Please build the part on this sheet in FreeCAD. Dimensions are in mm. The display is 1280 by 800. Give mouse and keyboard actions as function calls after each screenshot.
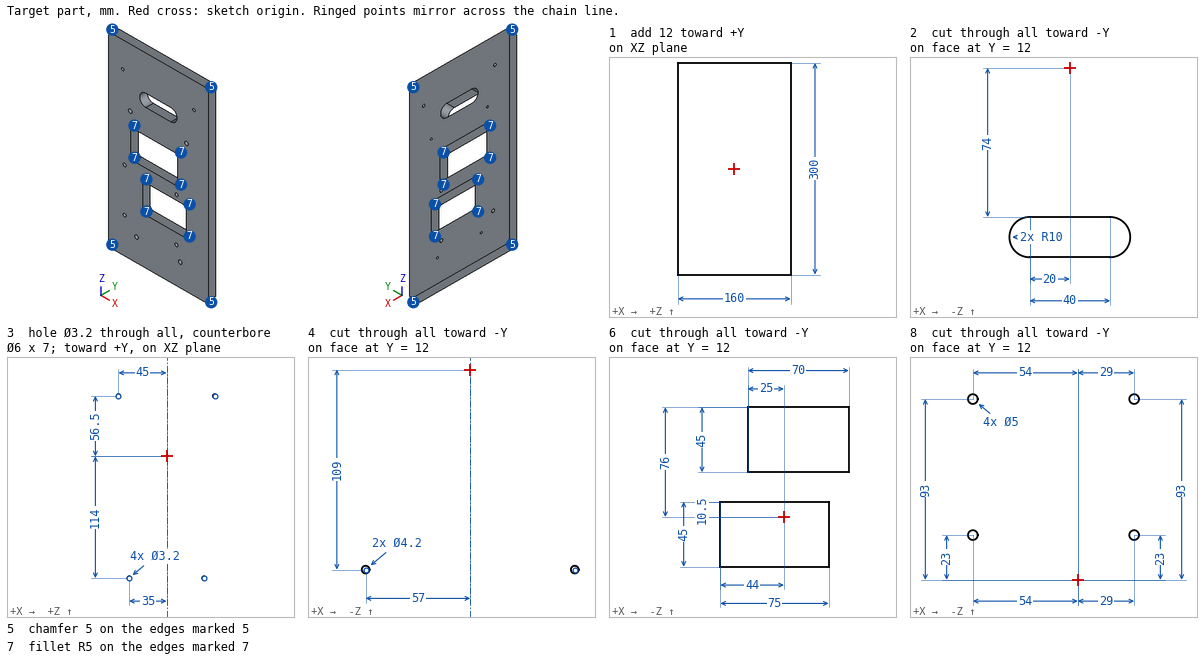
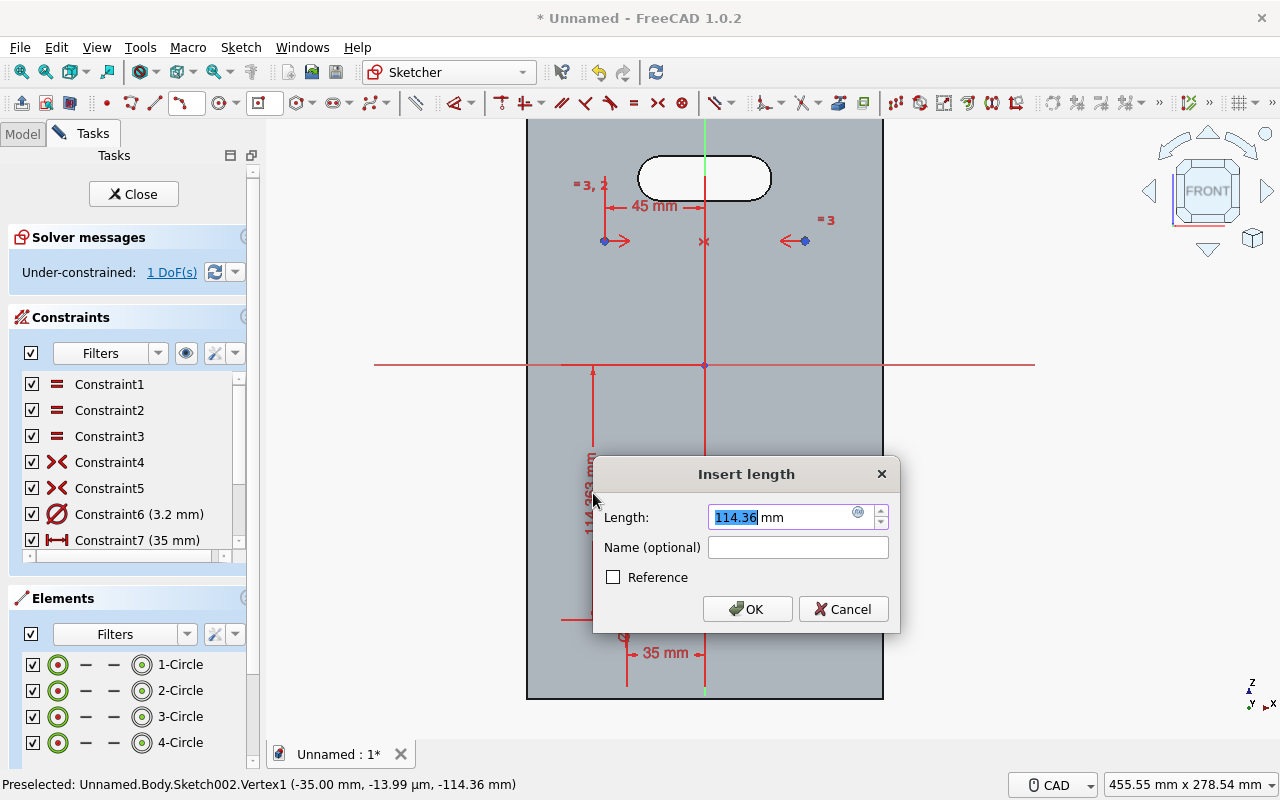
text(114)
key(Return)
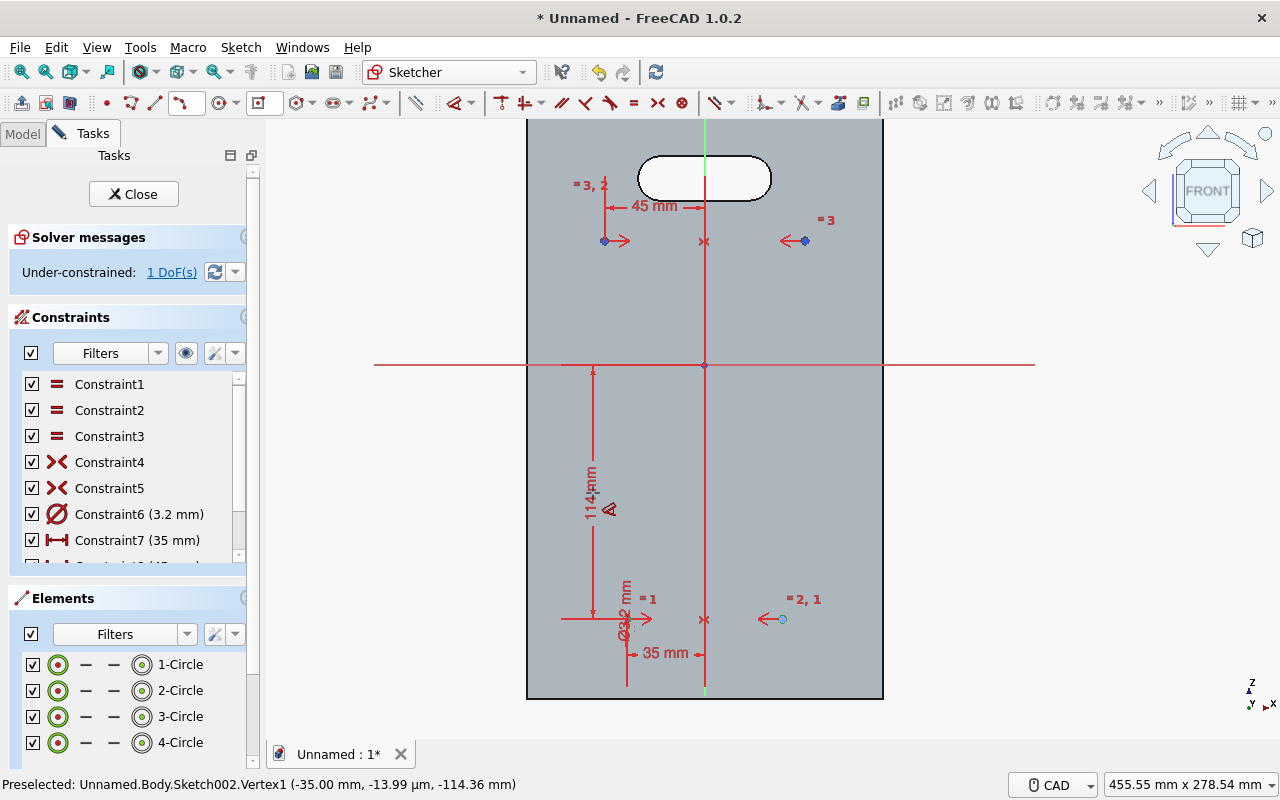
click(605, 241)
click(571, 303)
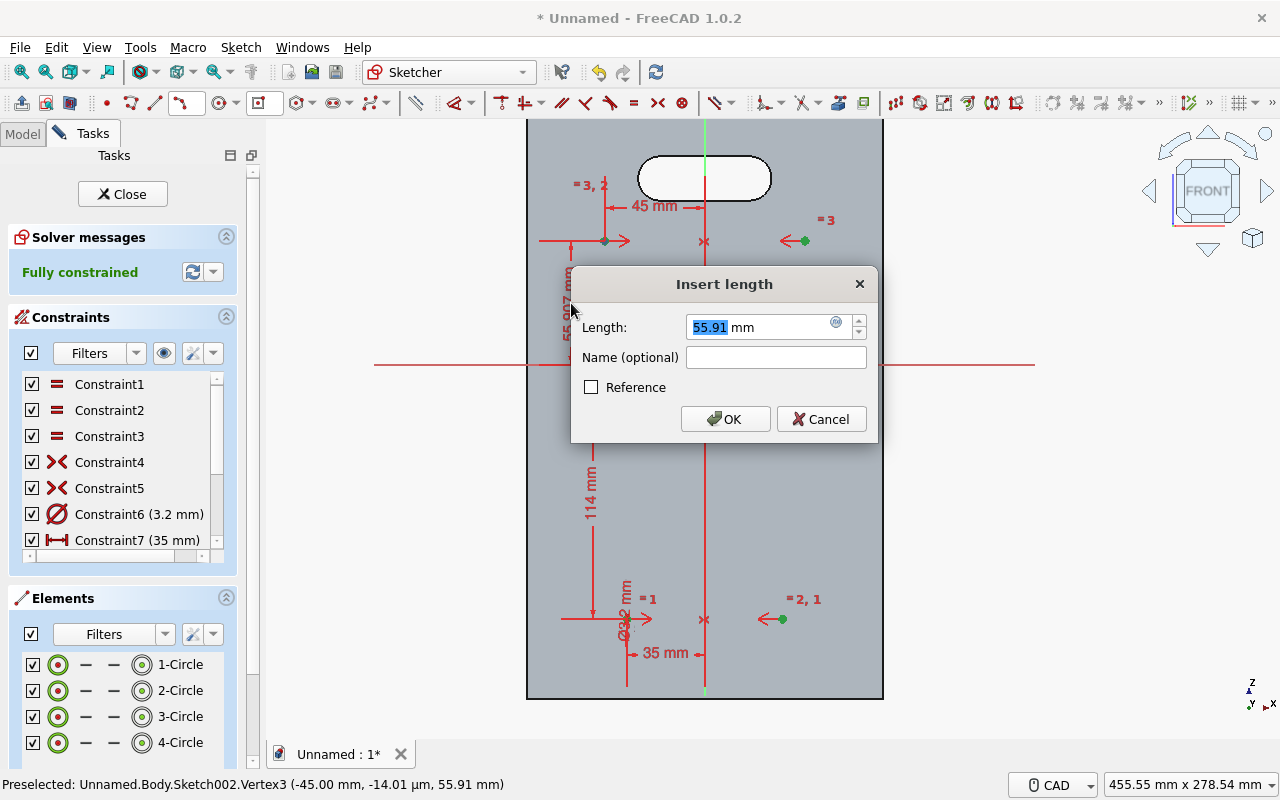
text(56.5)
key(Return)
key(Escape)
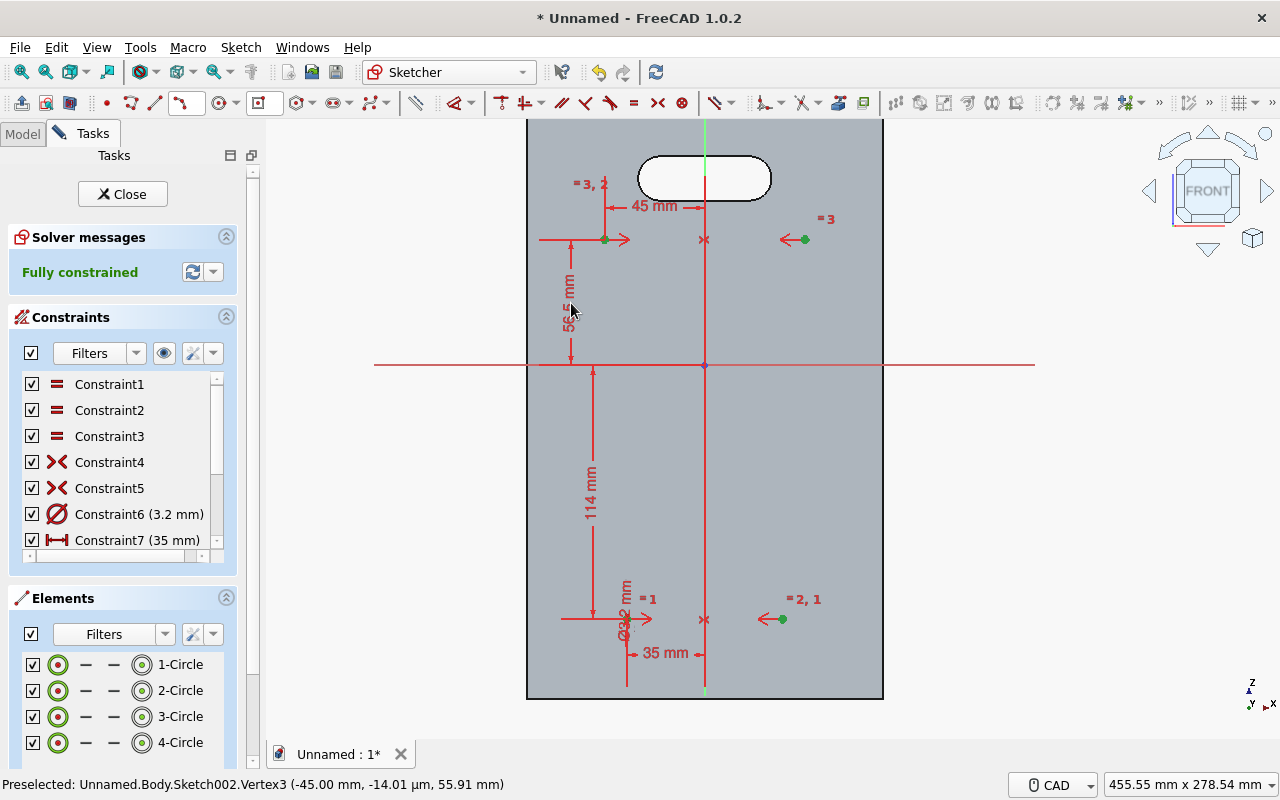
click(123, 194)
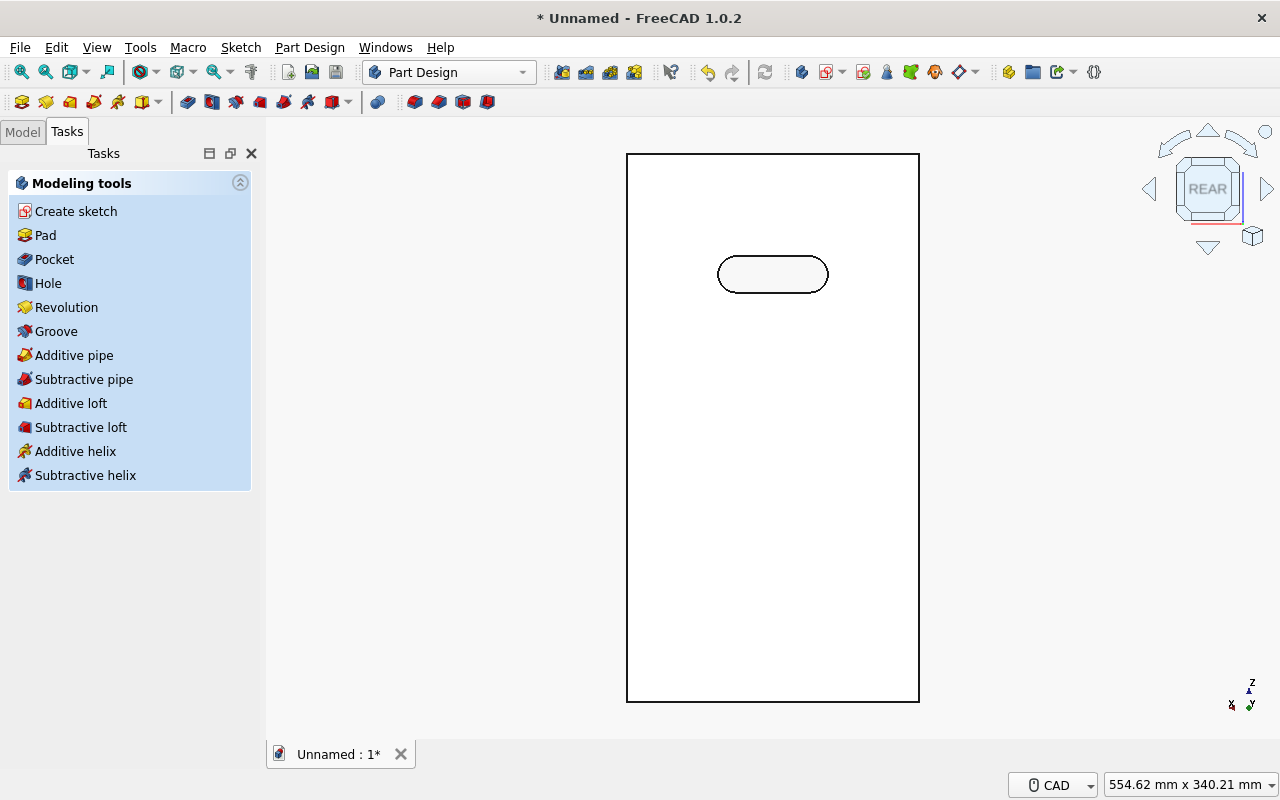
click(212, 102)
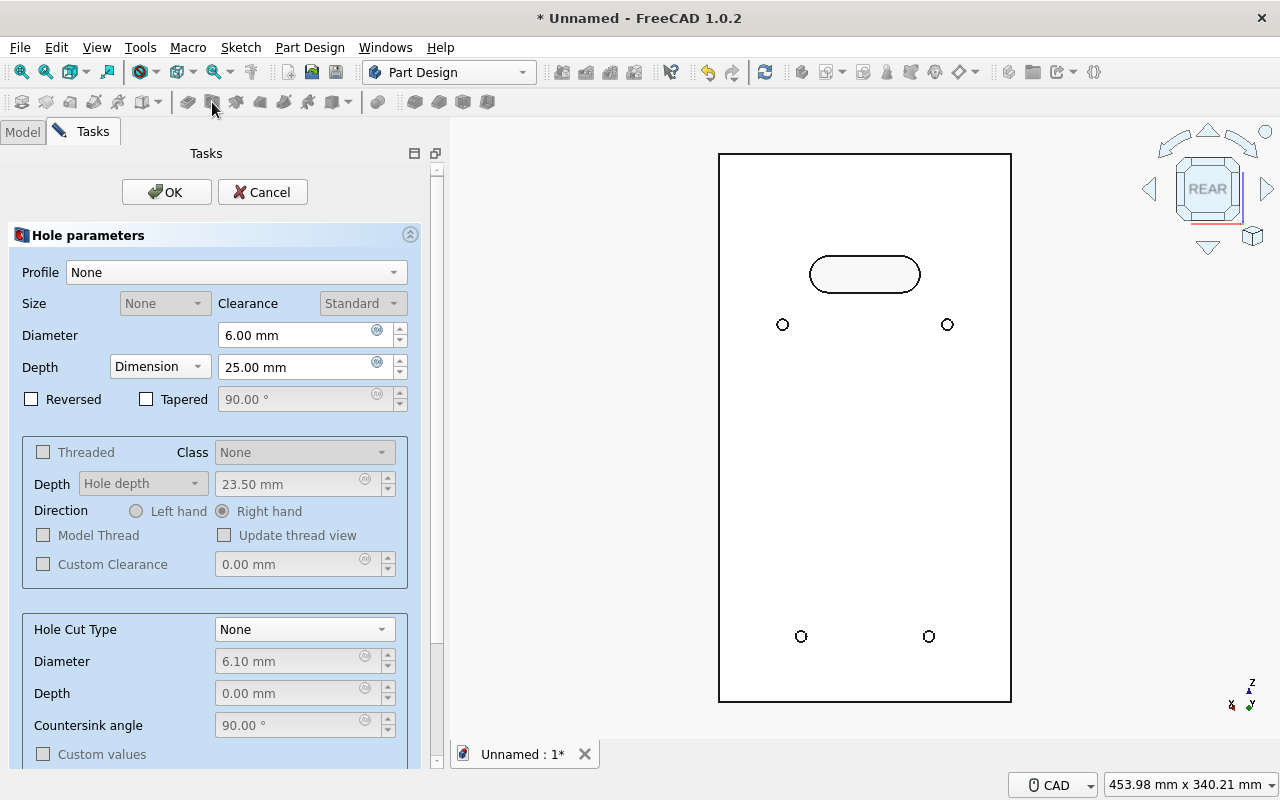
triple_click(305, 335)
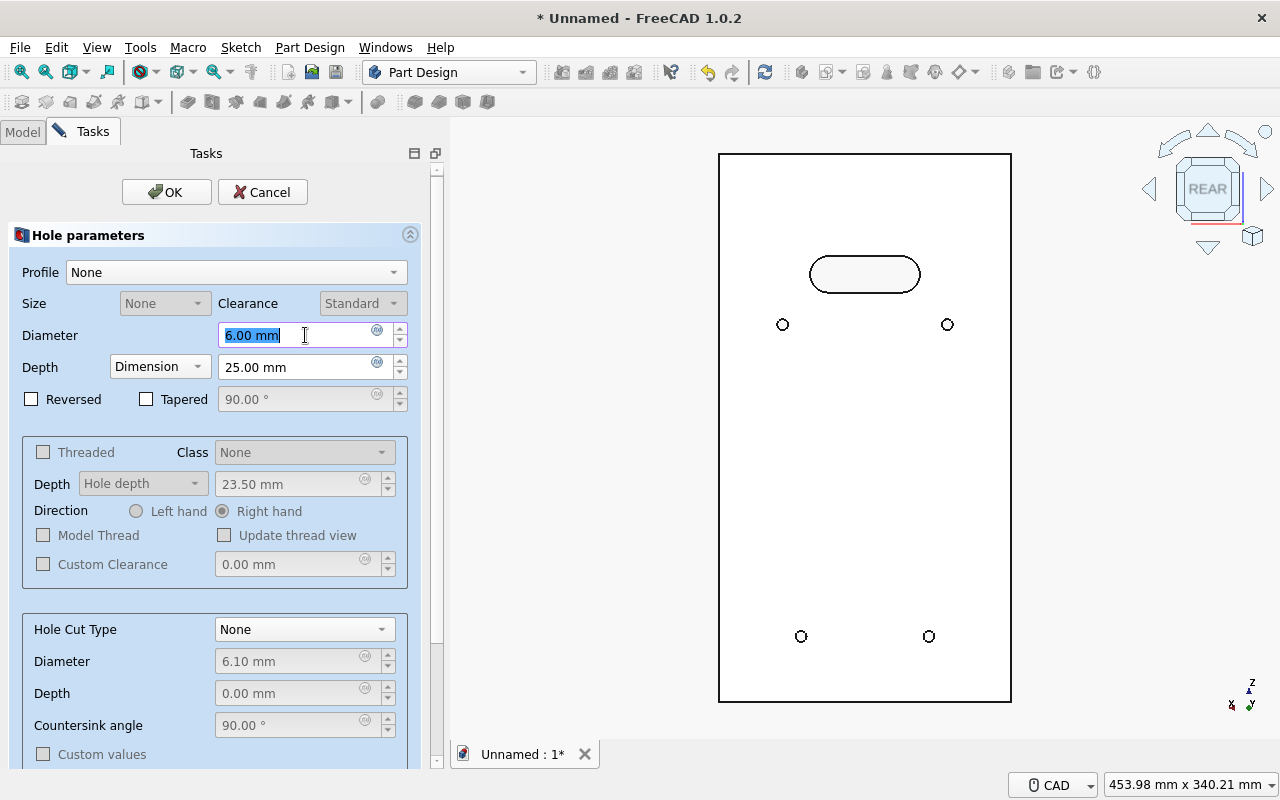
text(3.2)
key(Tab)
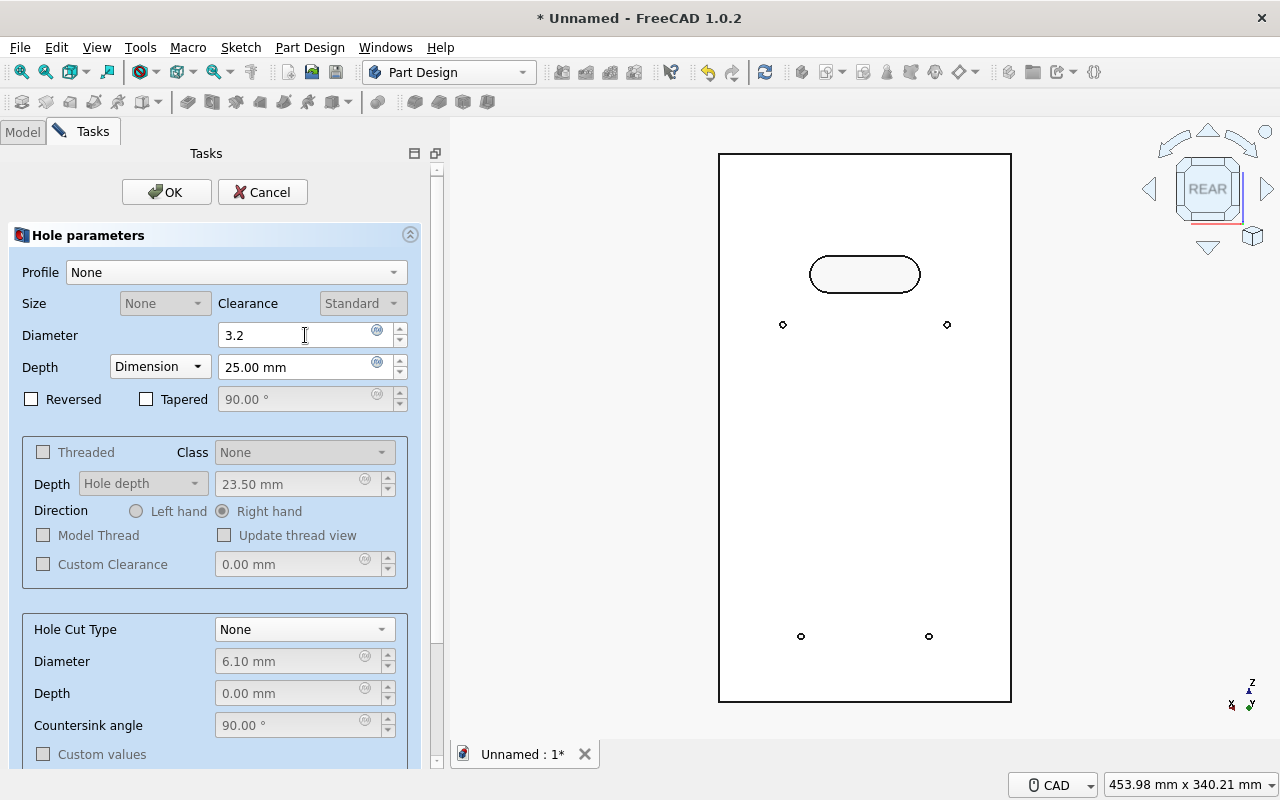
click(161, 366)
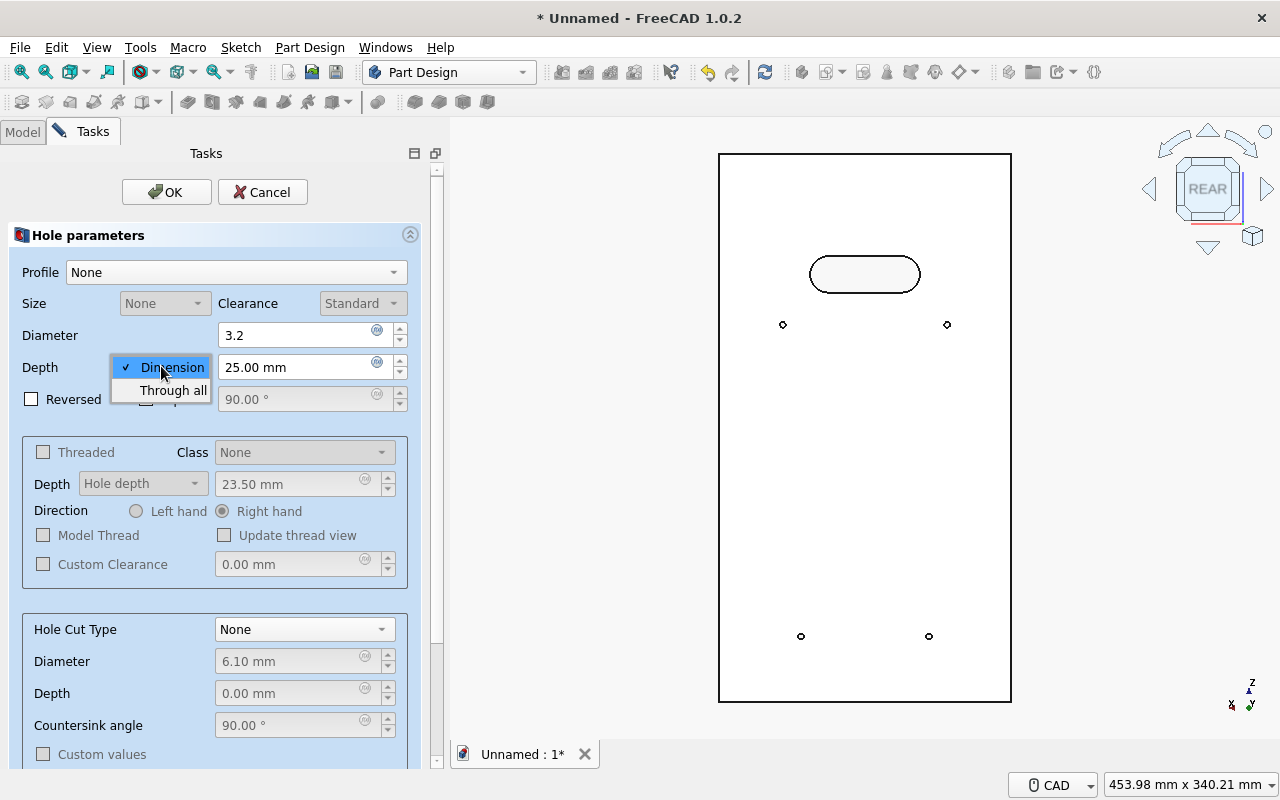
click(160, 390)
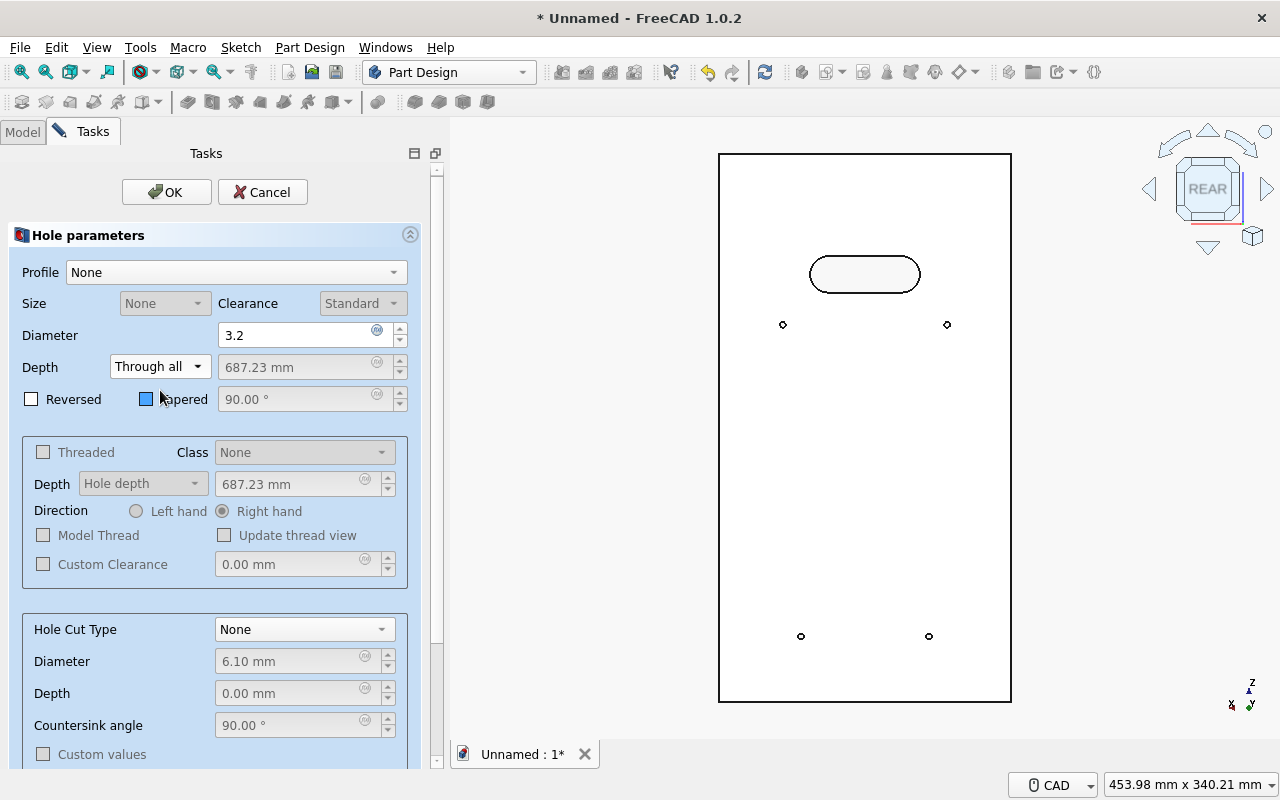
click(306, 630)